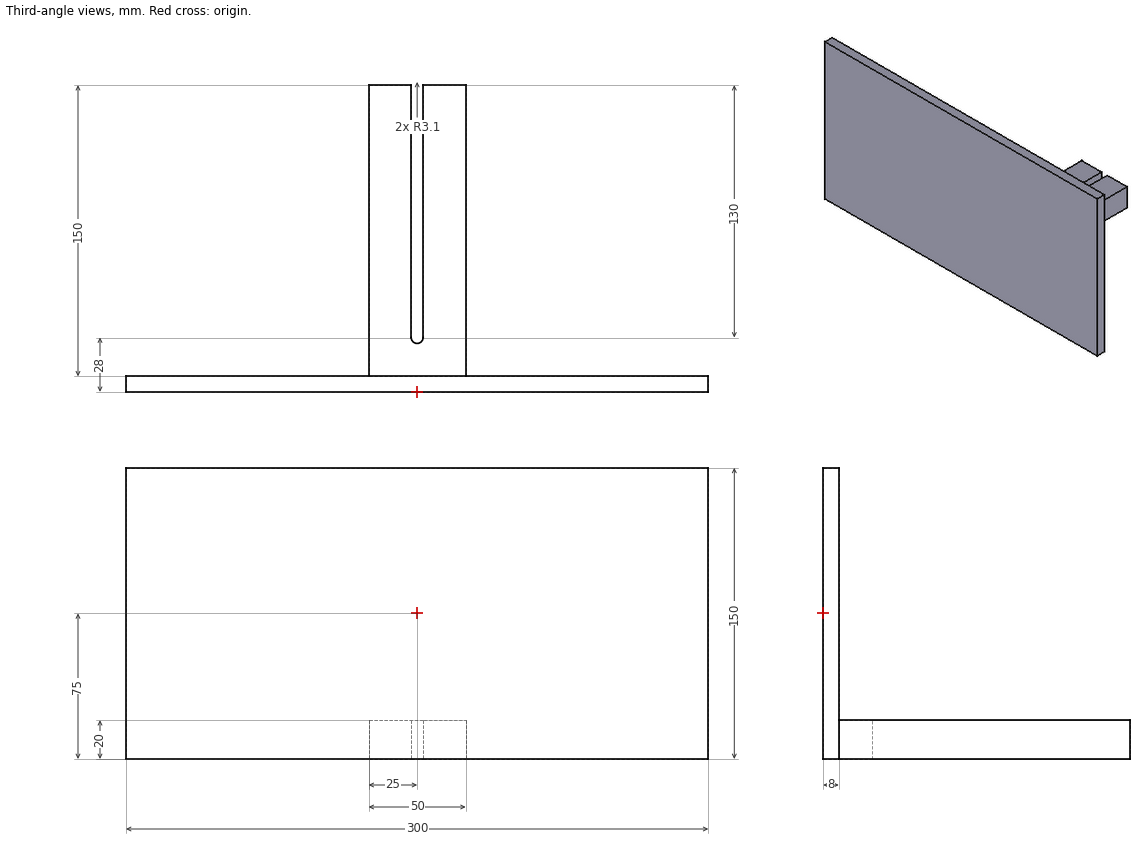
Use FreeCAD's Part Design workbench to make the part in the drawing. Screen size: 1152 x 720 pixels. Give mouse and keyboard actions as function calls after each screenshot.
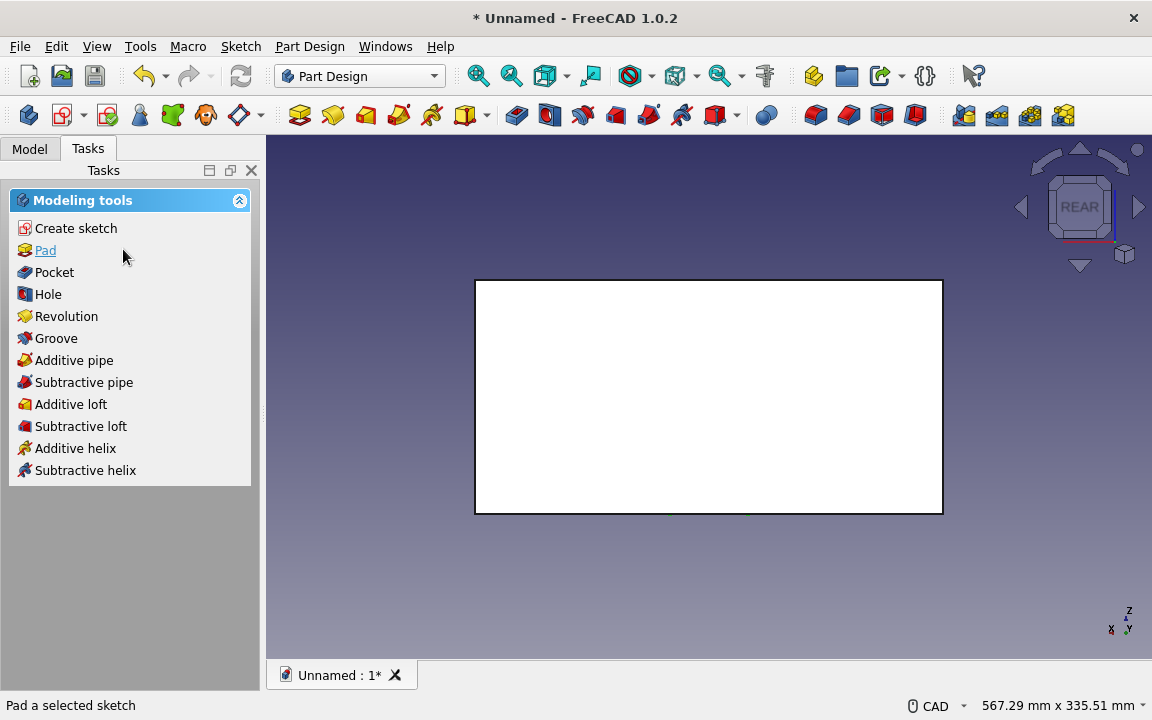
click(300, 116)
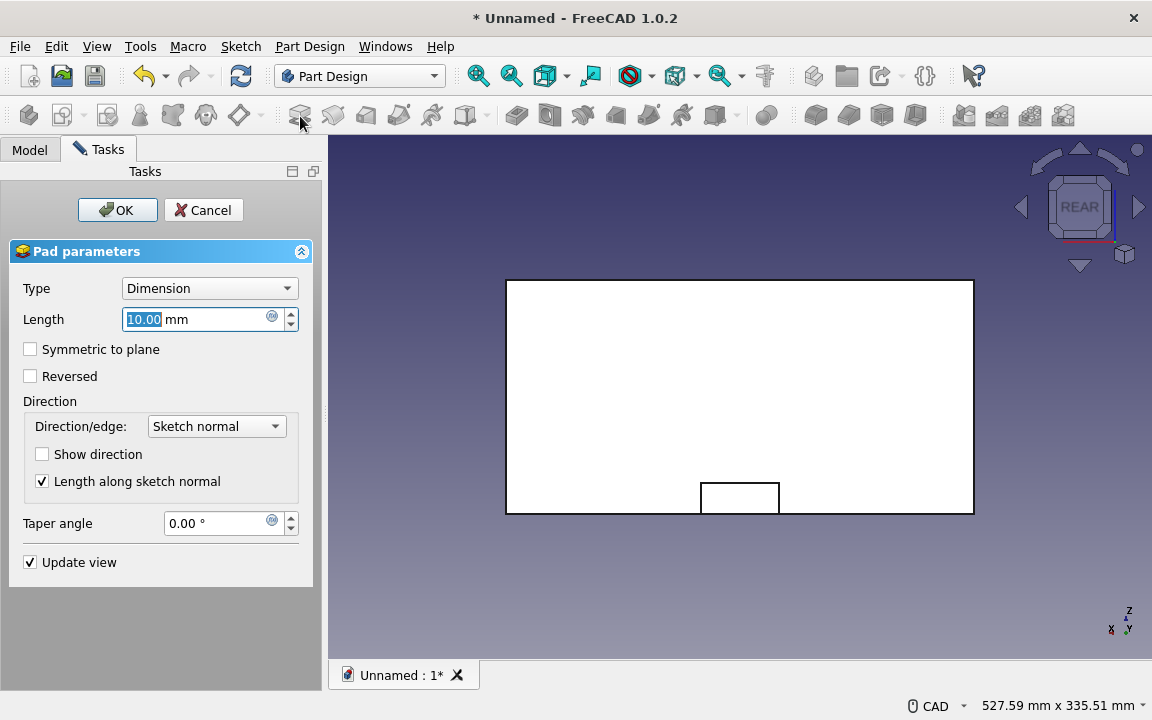
text(150)
key(Tab)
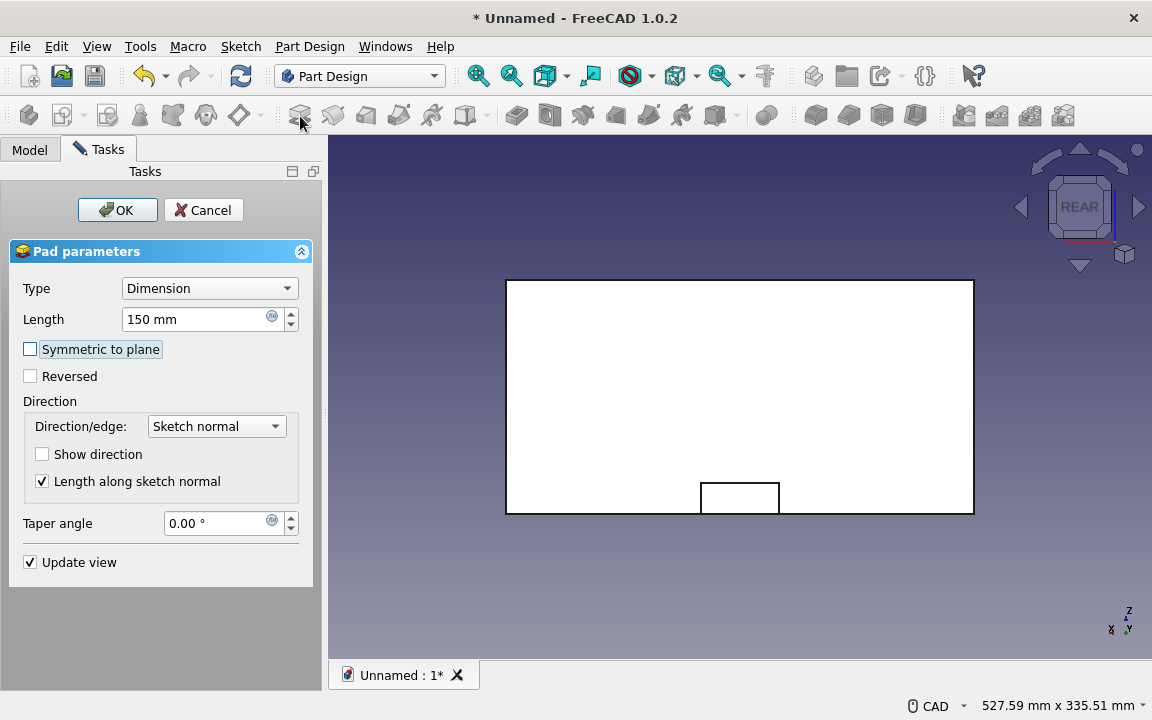
click(118, 210)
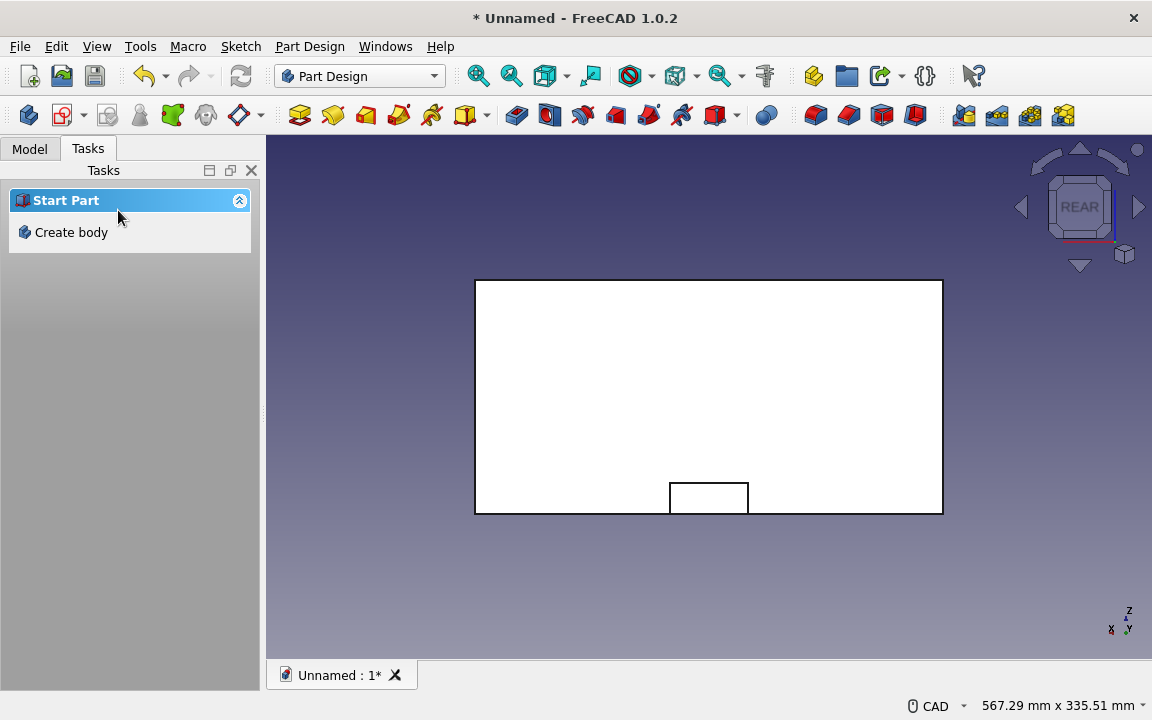
key(0)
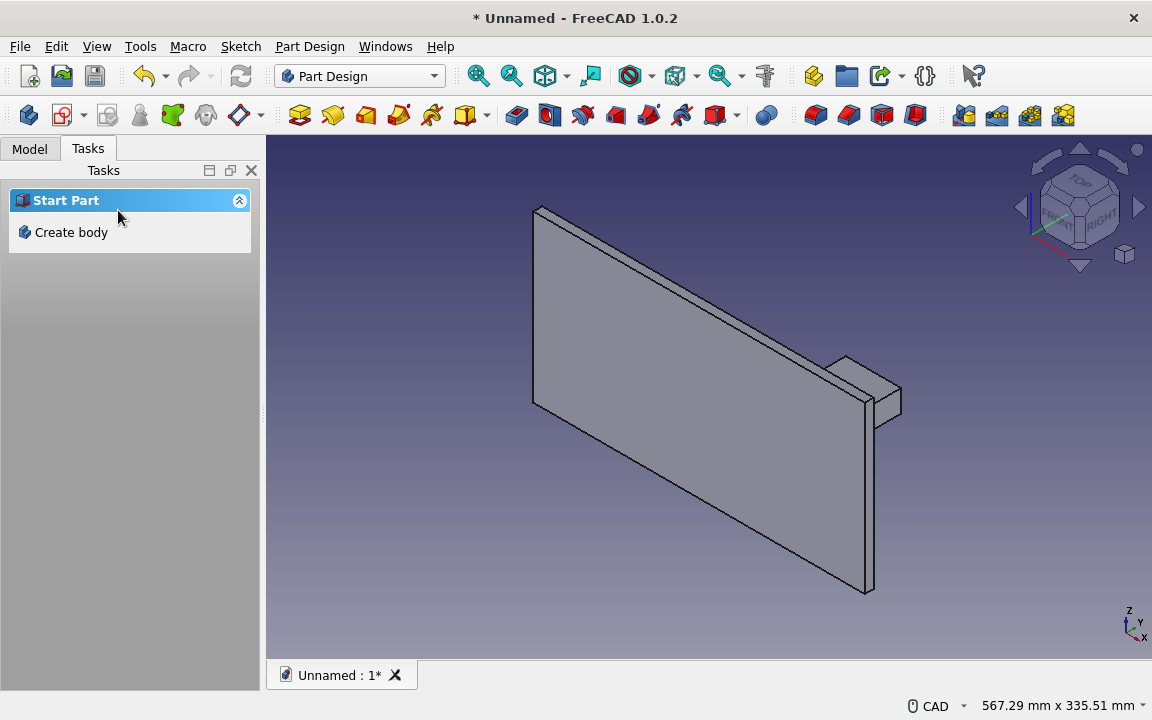
click(479, 76)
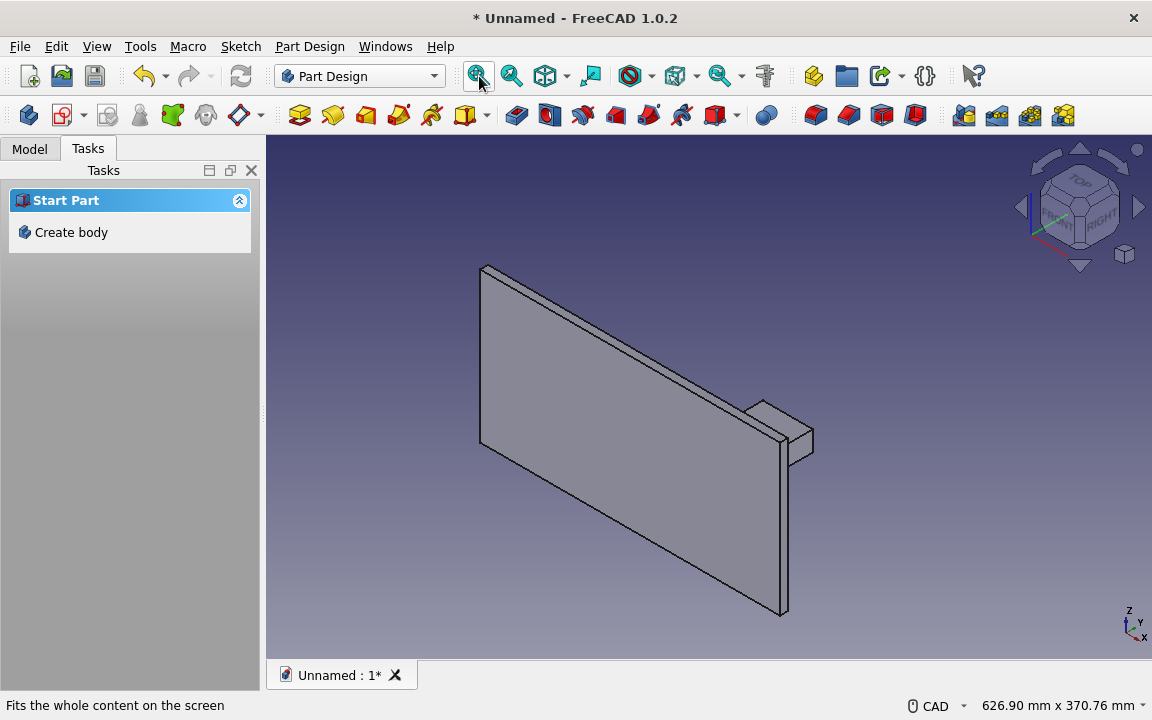
key(2)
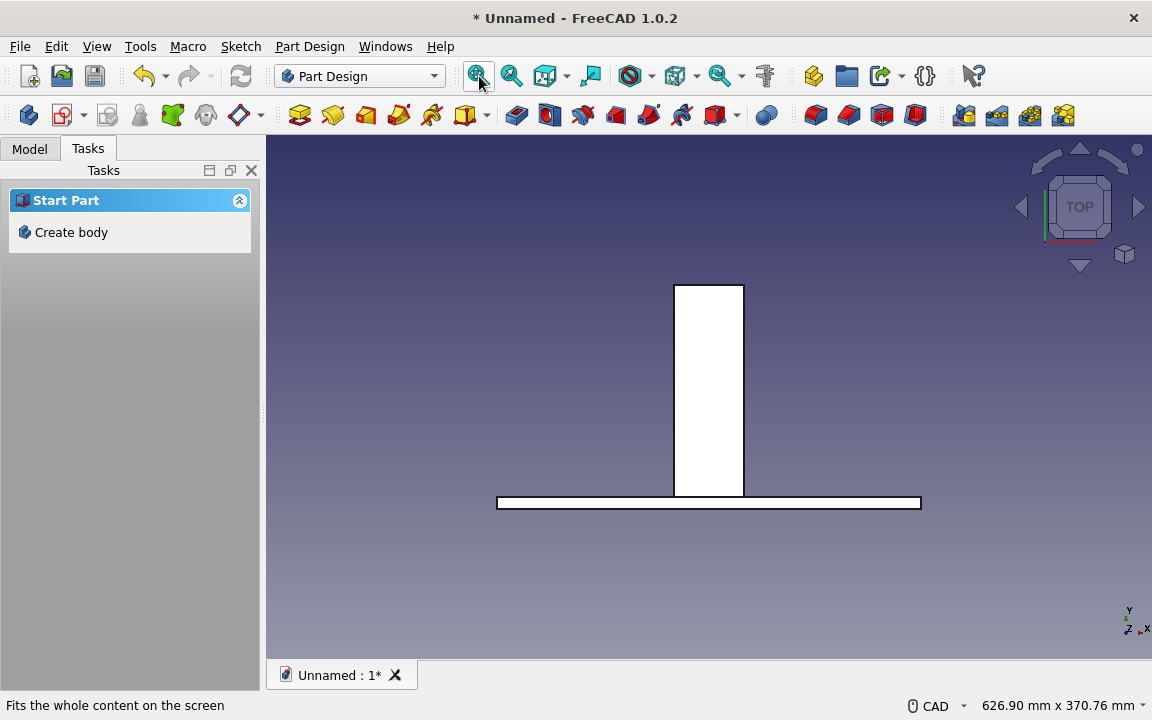
click(709, 330)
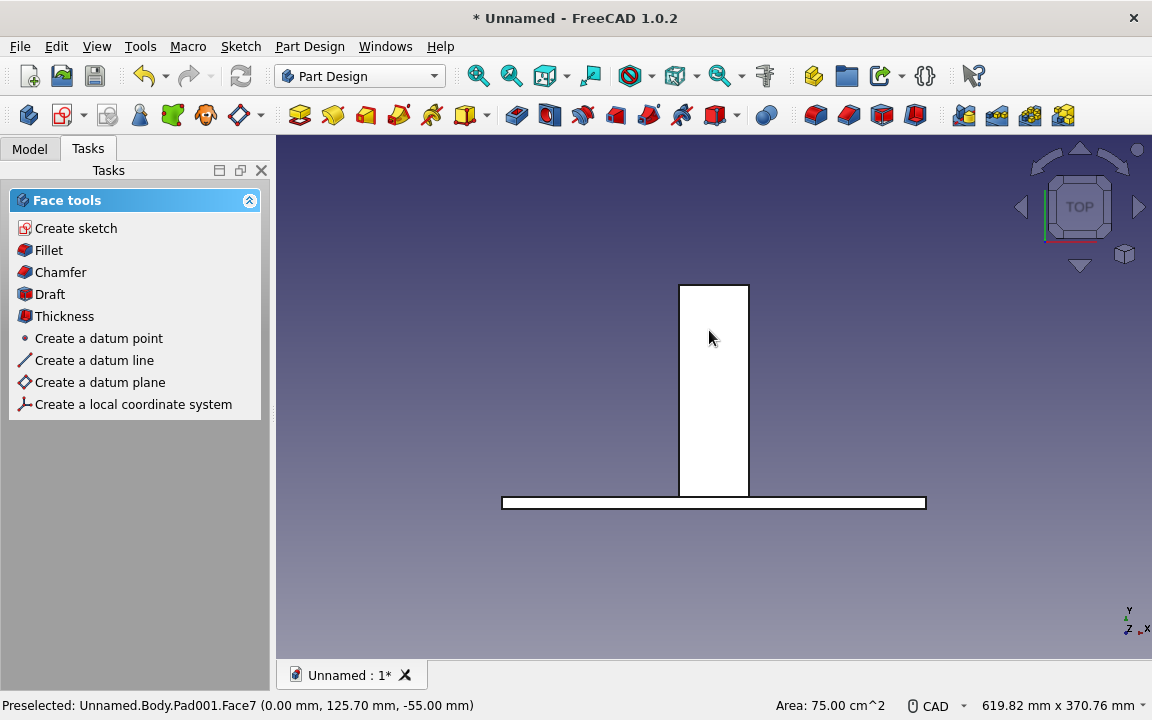
click(62, 116)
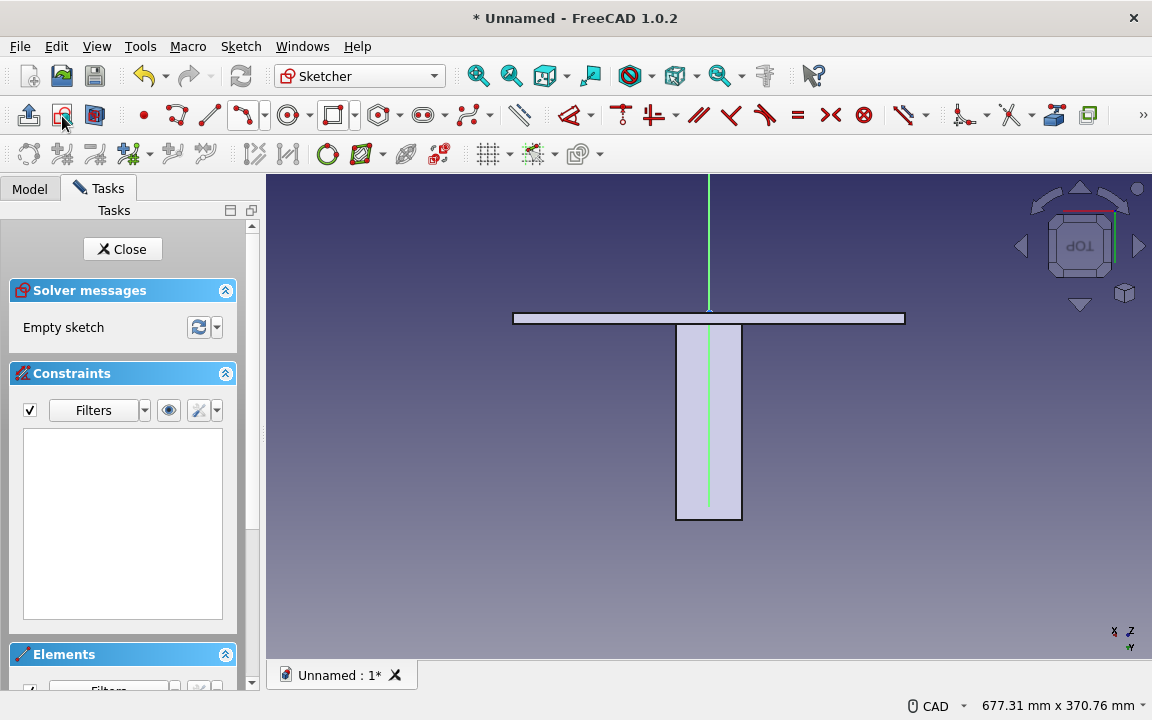
click(95, 116)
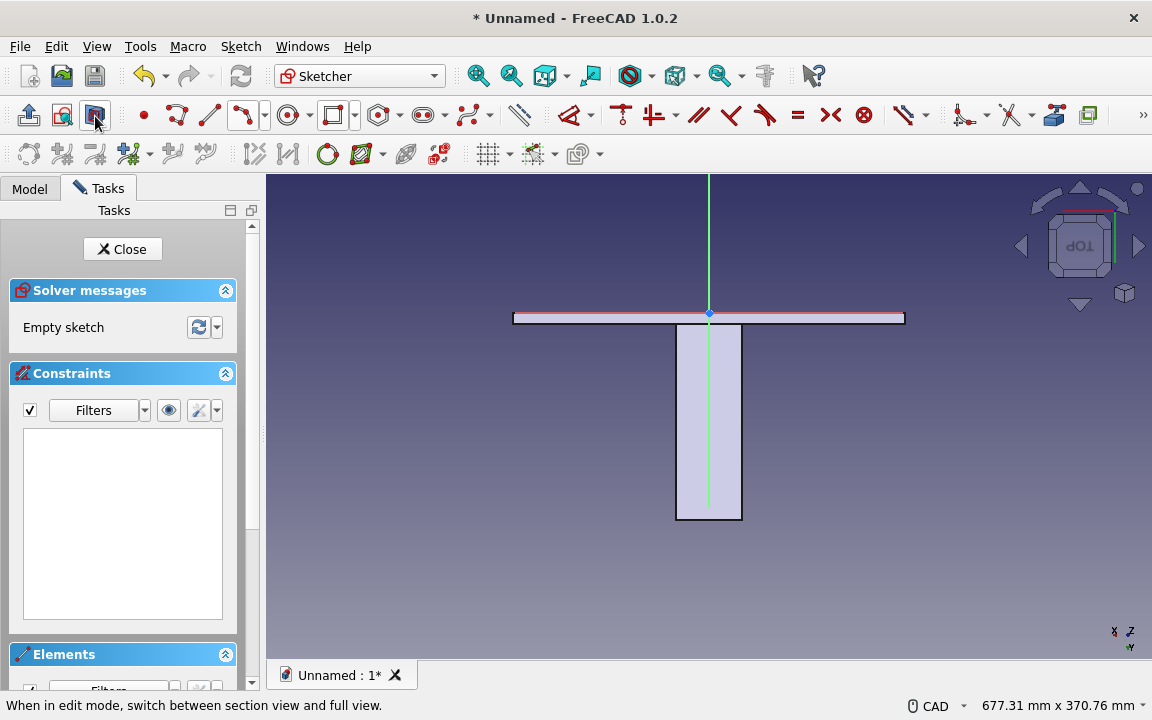
scroll(848, 423, up, 2)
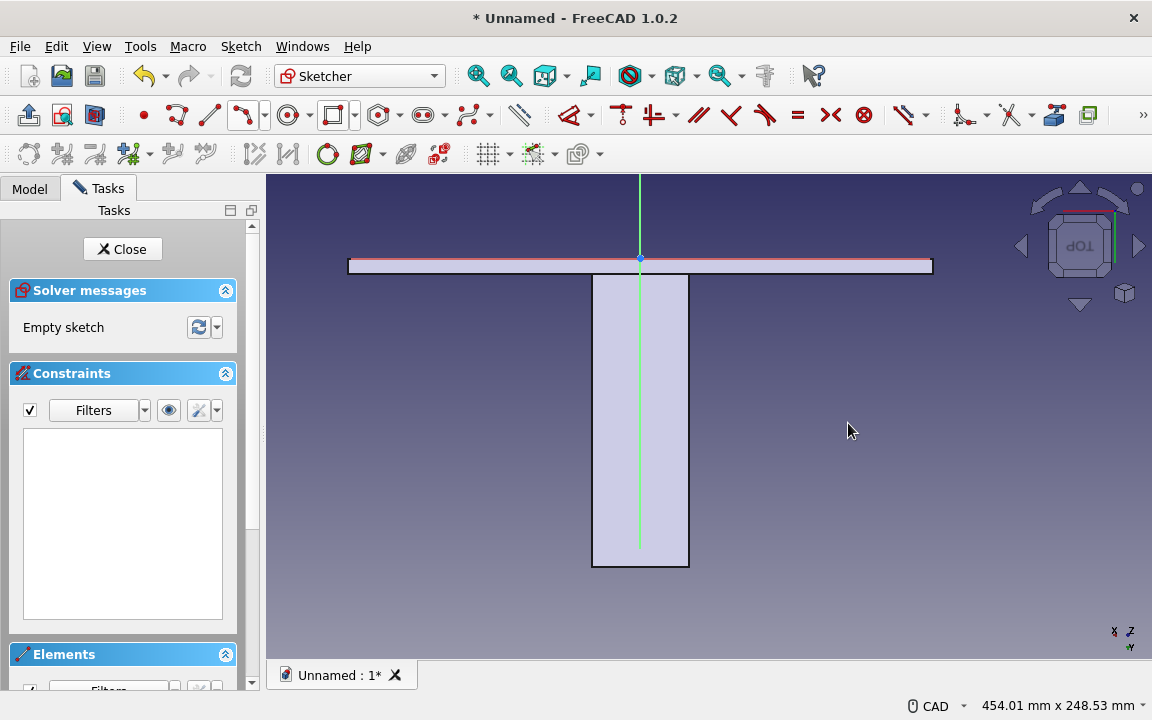
click(422, 116)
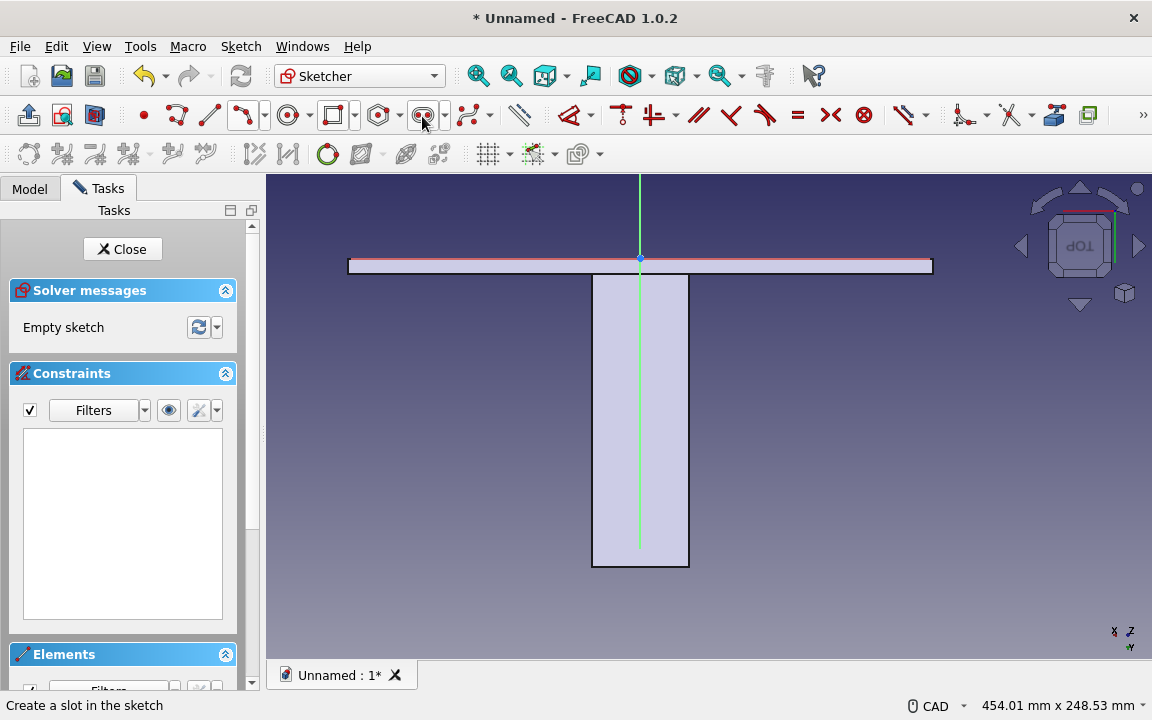
scroll(640, 567, up, 7)